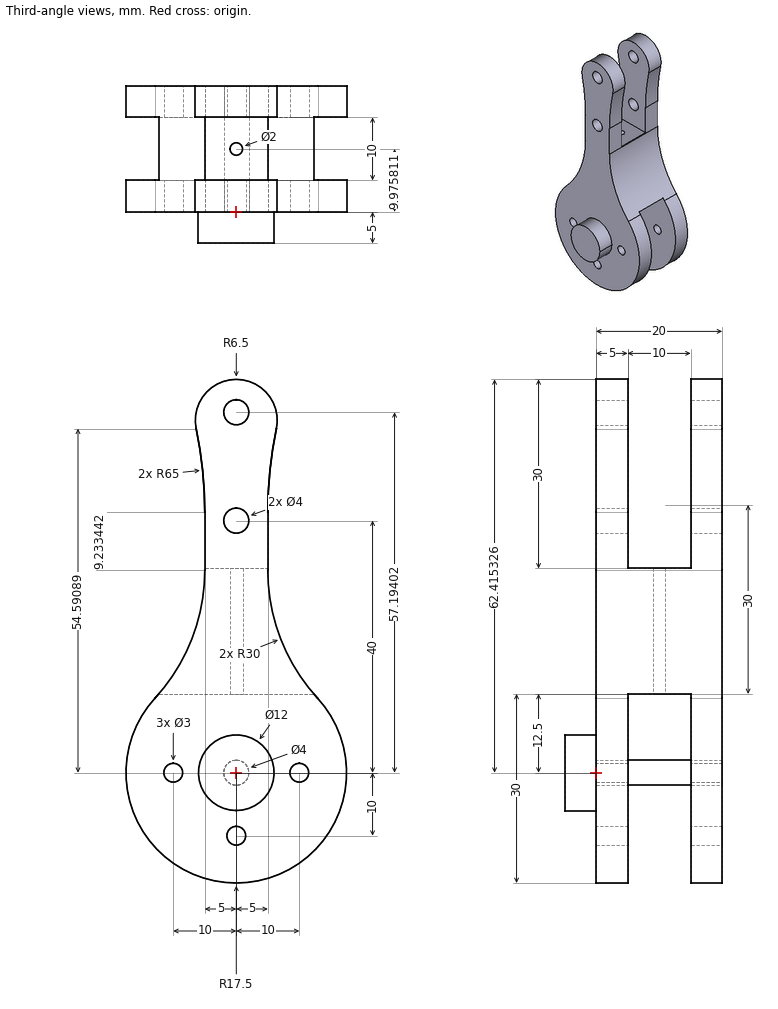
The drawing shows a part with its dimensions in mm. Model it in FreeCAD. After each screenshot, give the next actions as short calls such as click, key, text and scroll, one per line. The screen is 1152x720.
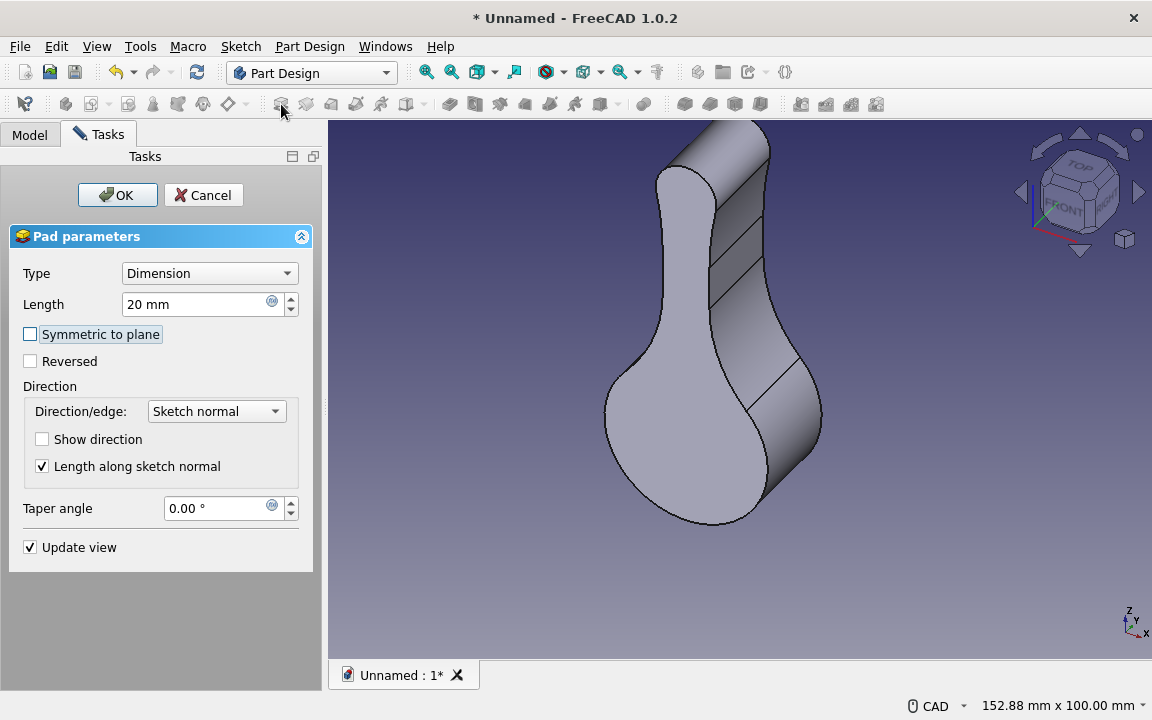
click(31, 361)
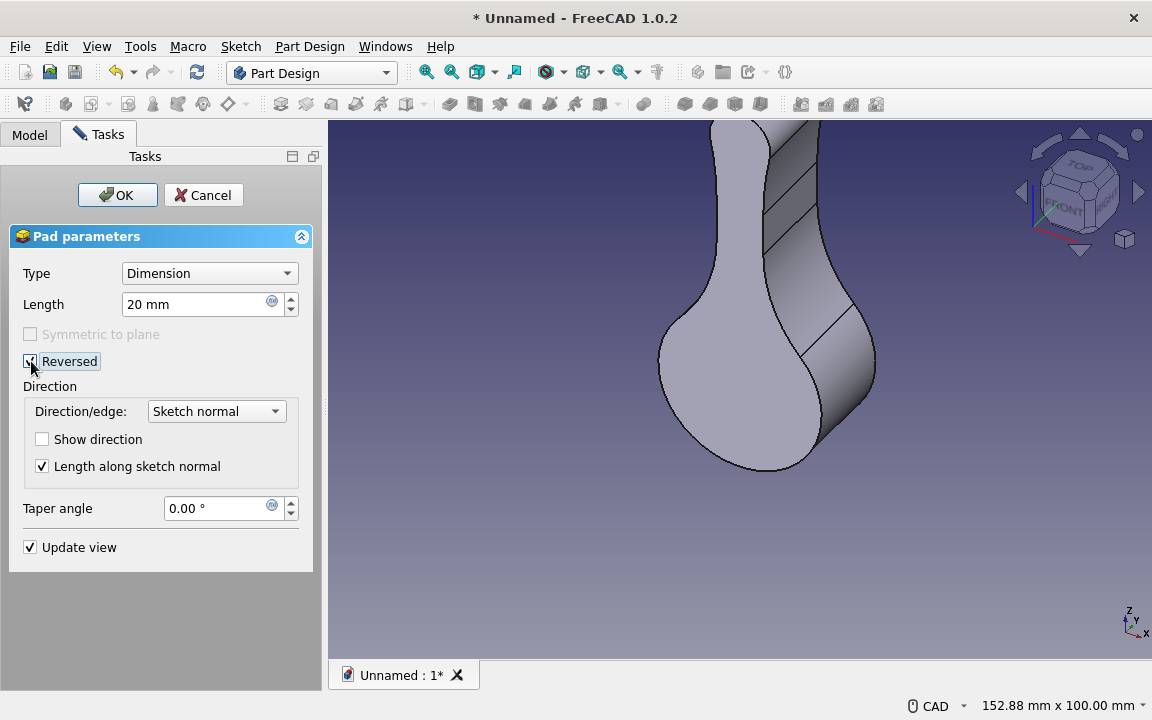
click(118, 195)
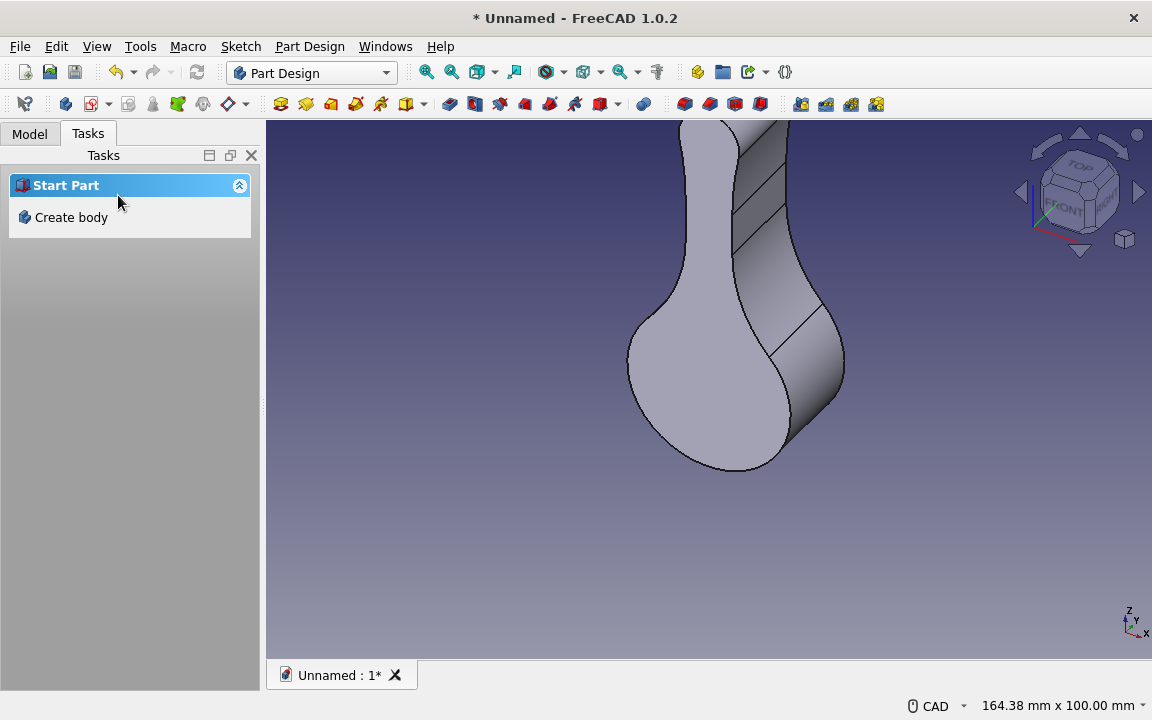
key(v)
key(f)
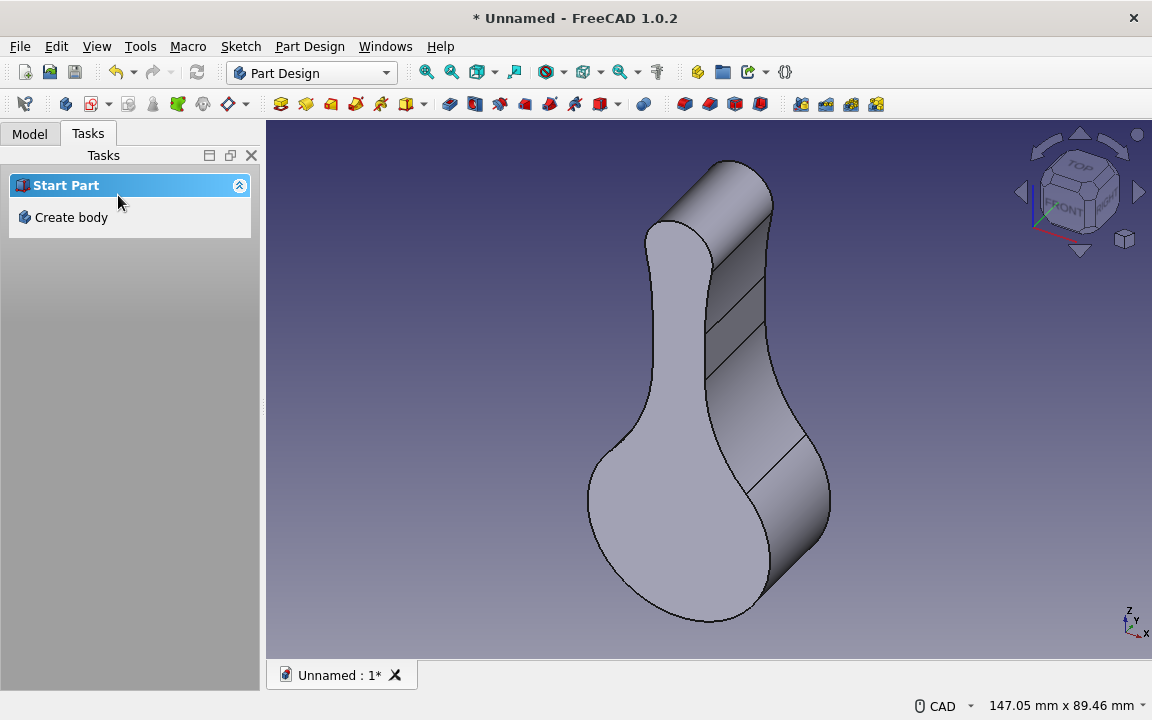
key(4)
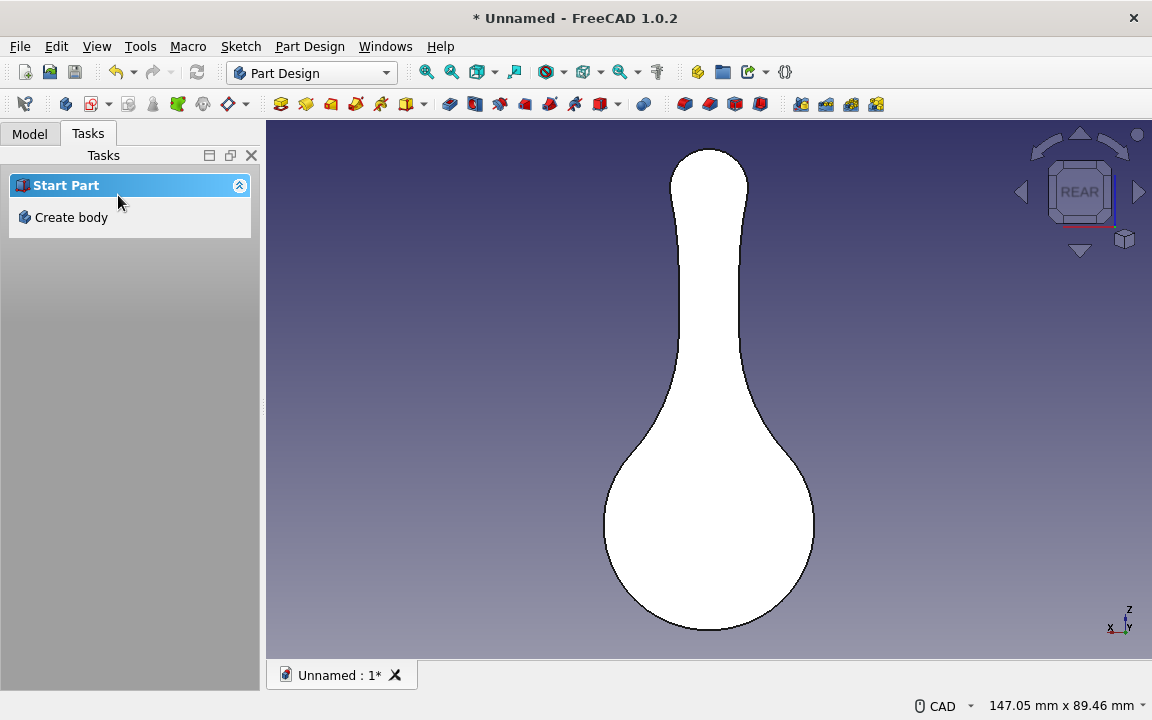
click(709, 526)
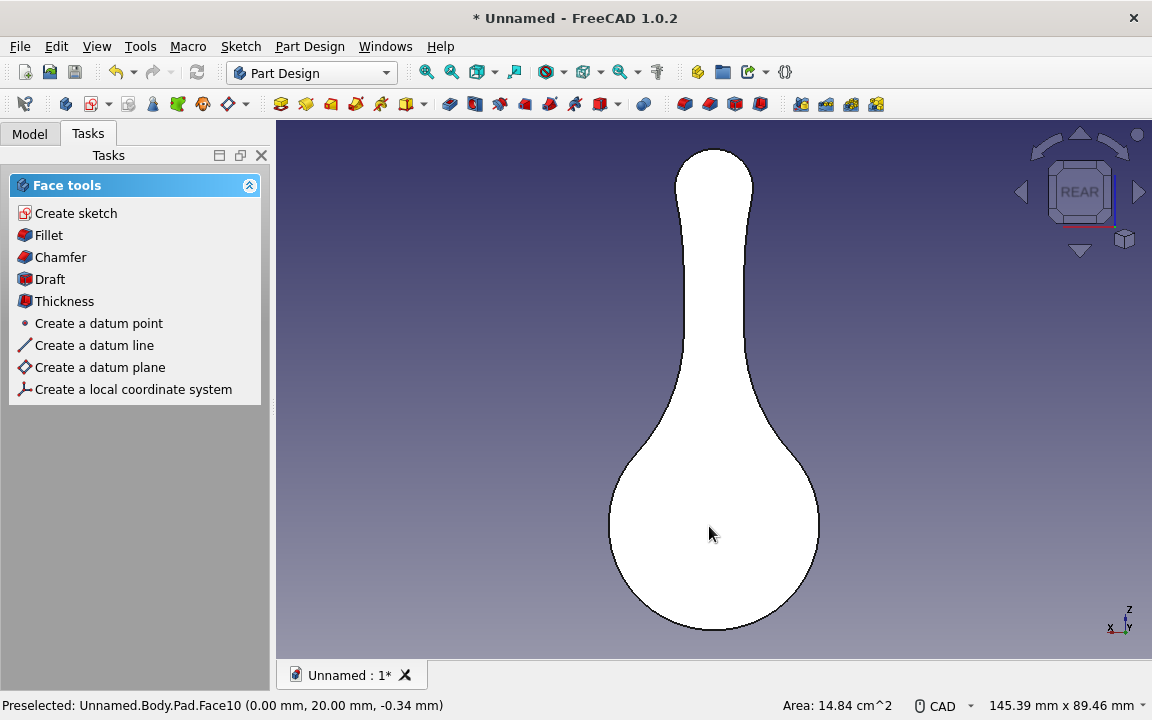
click(90, 104)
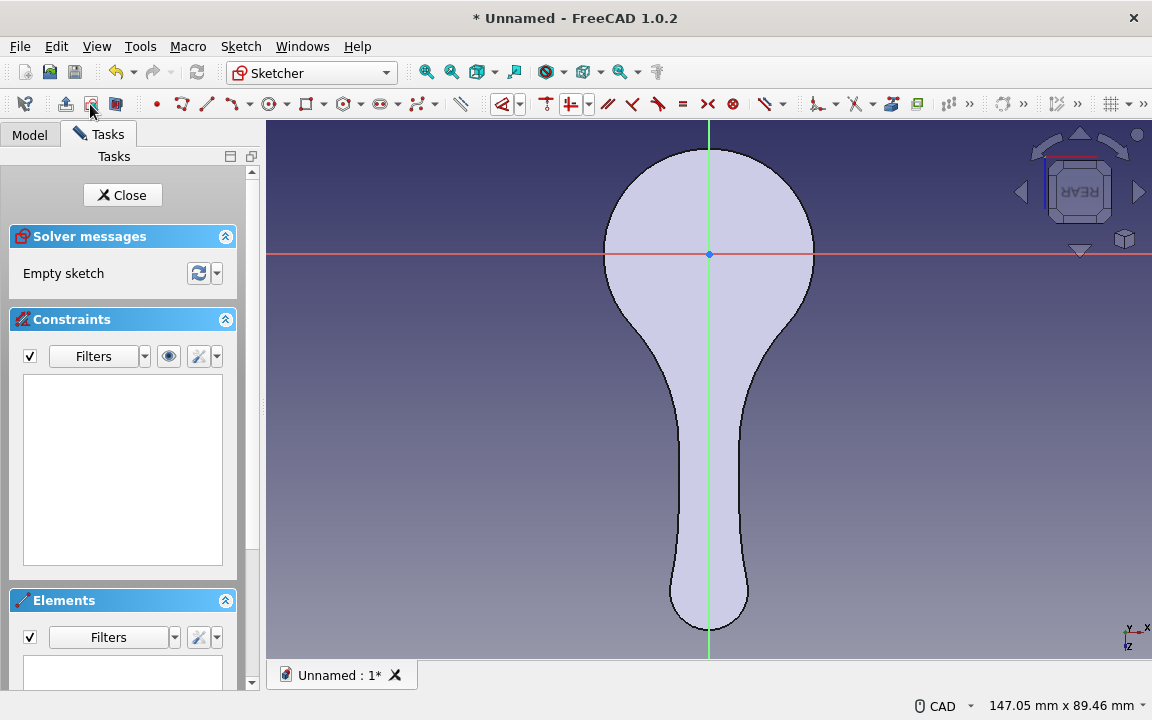
scroll(749, 631, up, 5)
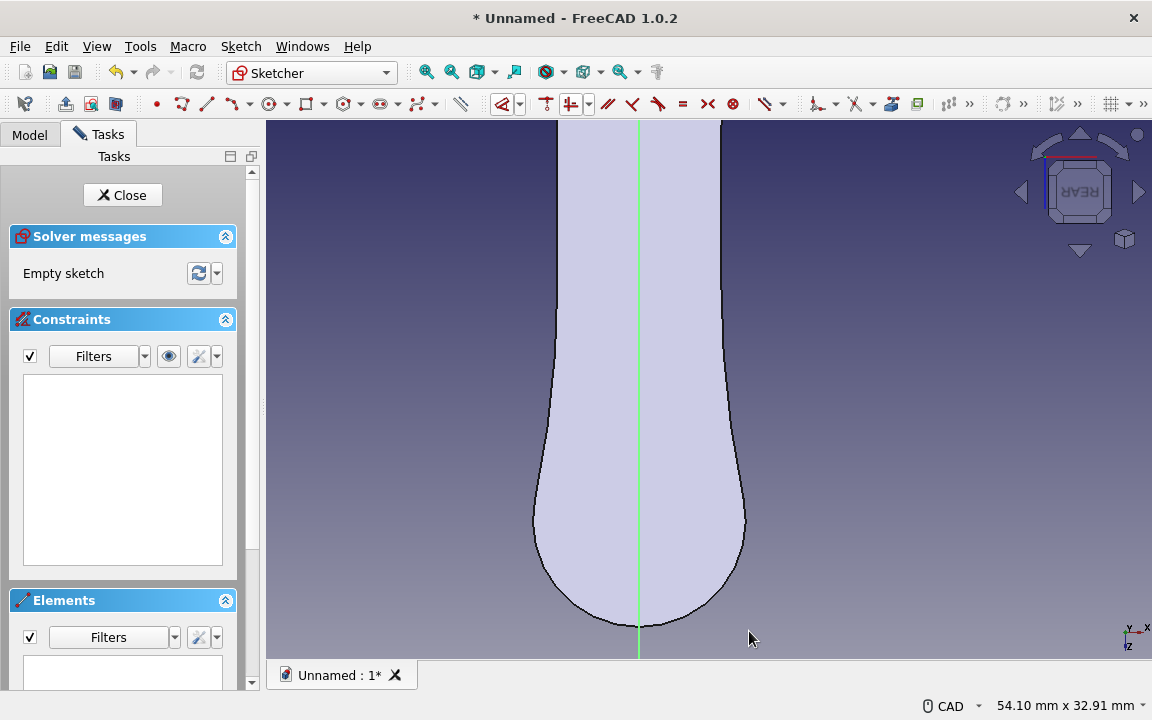
click(268, 104)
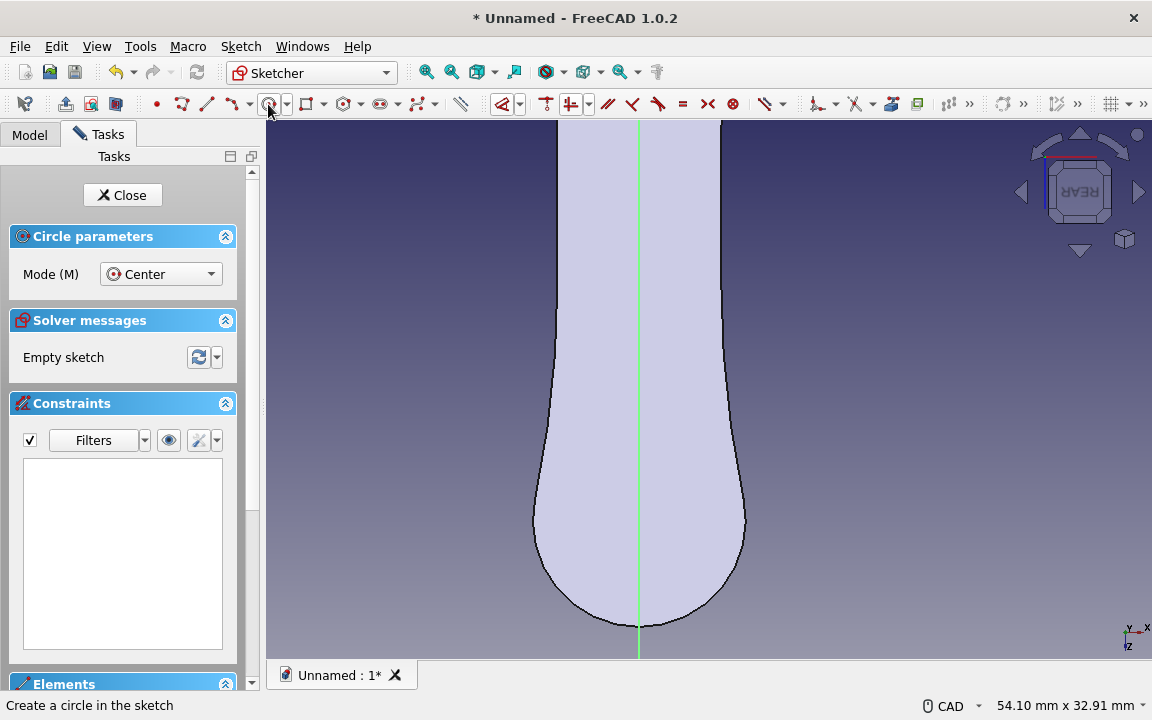
click(639, 260)
click(662, 237)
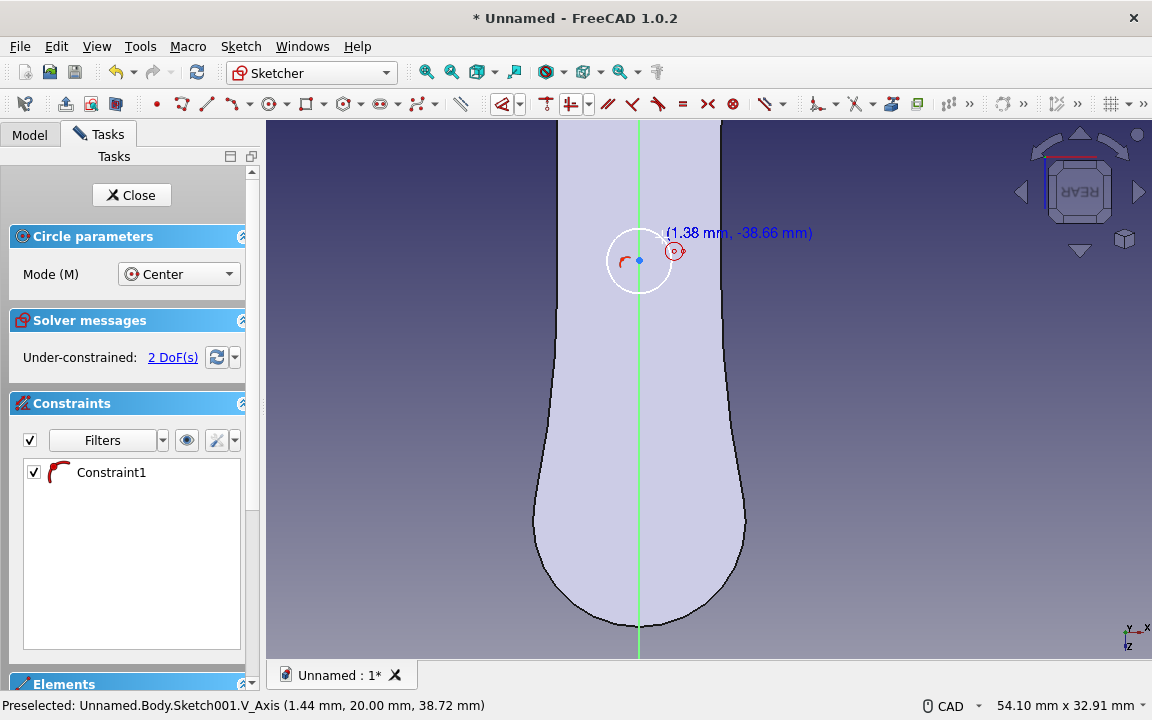
click(639, 541)
click(662, 518)
key(Escape)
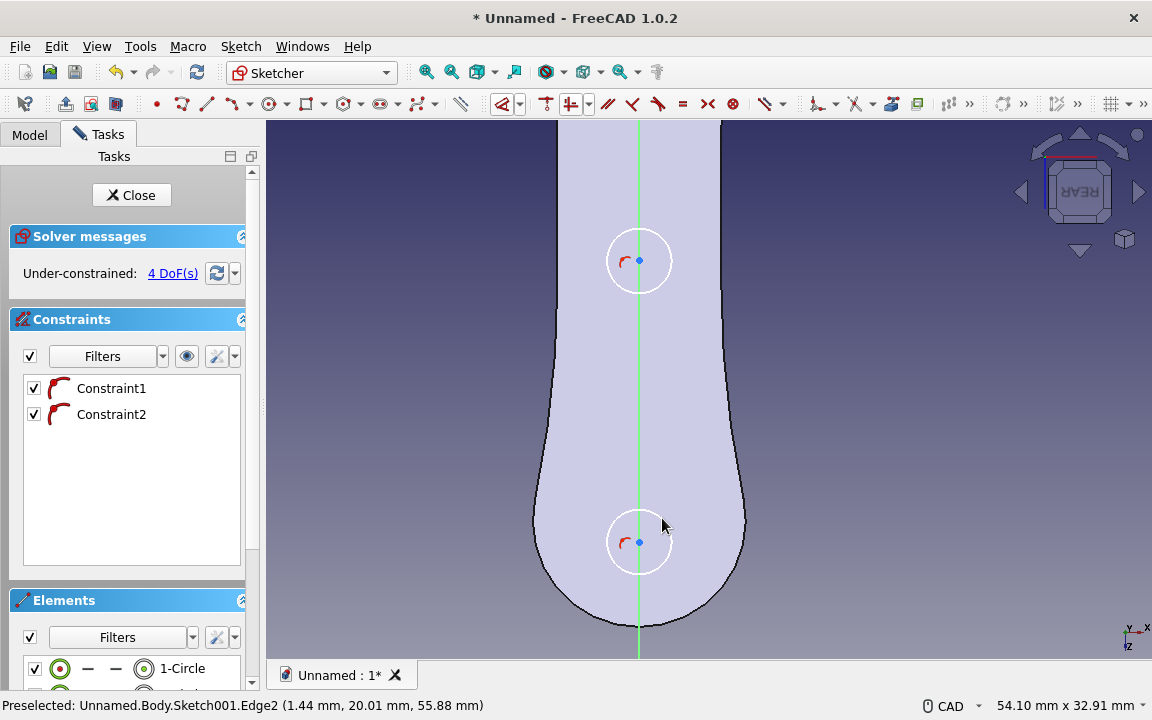
click(662, 238)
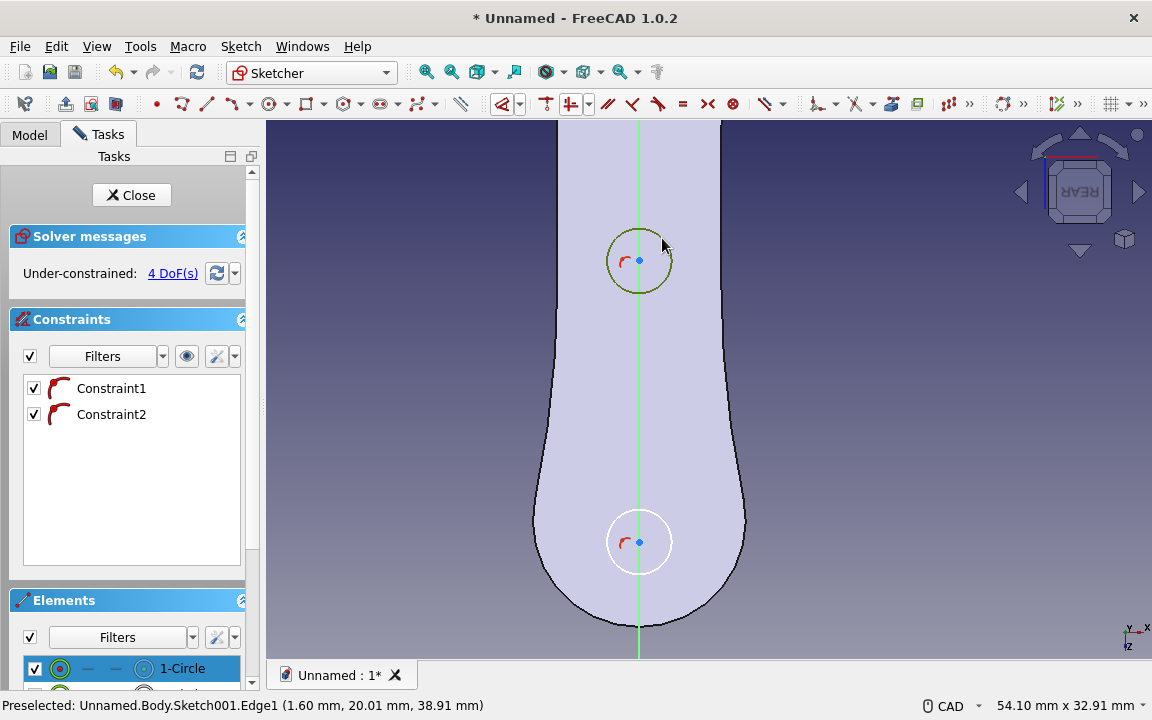
click(662, 519)